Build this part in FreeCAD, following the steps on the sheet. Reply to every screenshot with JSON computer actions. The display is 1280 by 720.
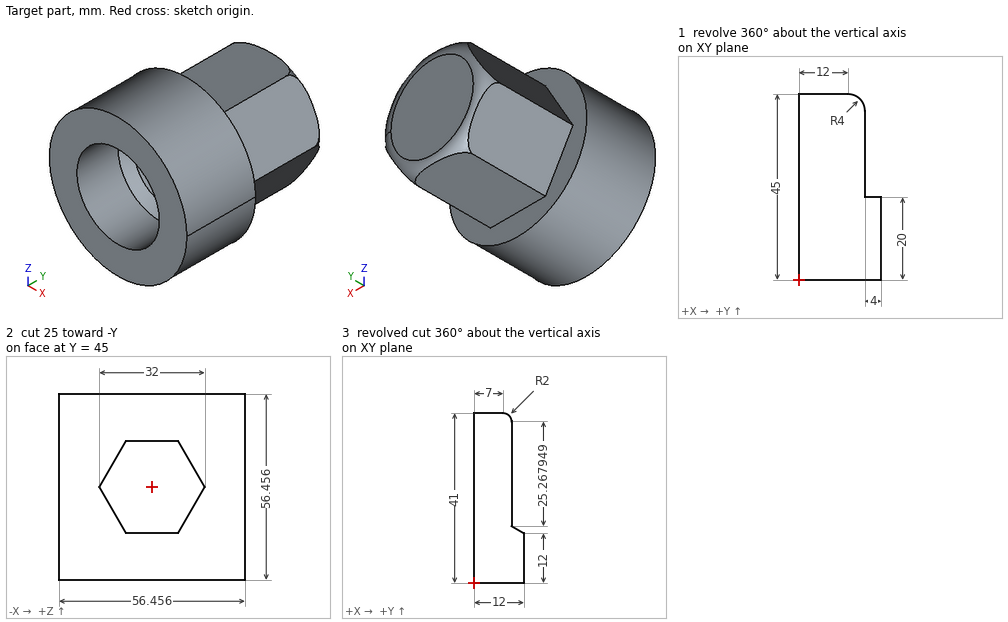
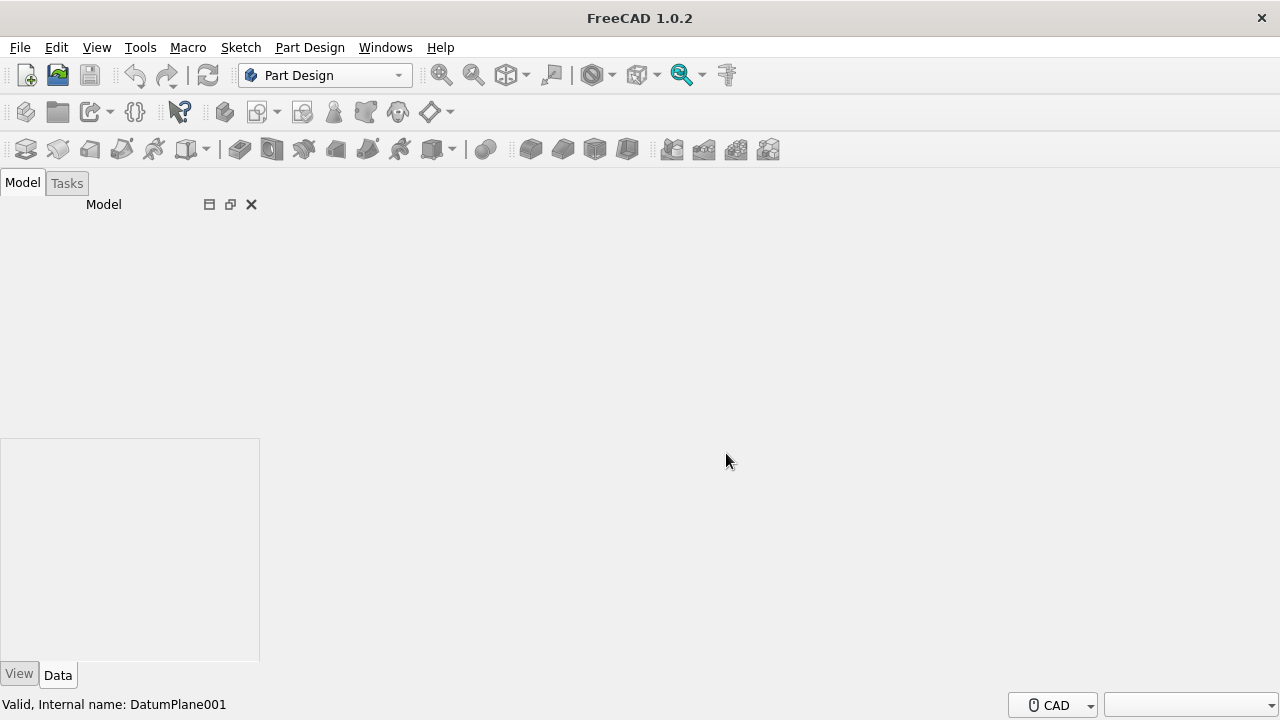
{"action": "key", "text": "ctrl+n"}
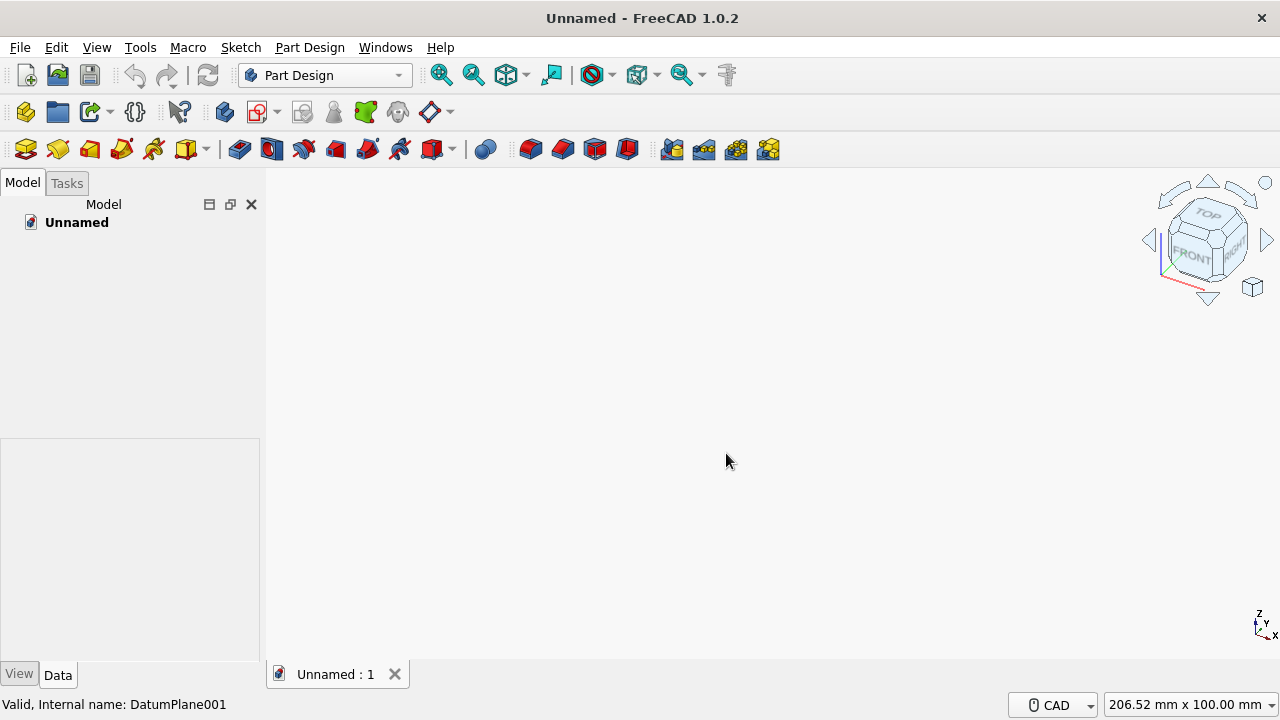
{"action": "left_click", "coordinate": [258, 112]}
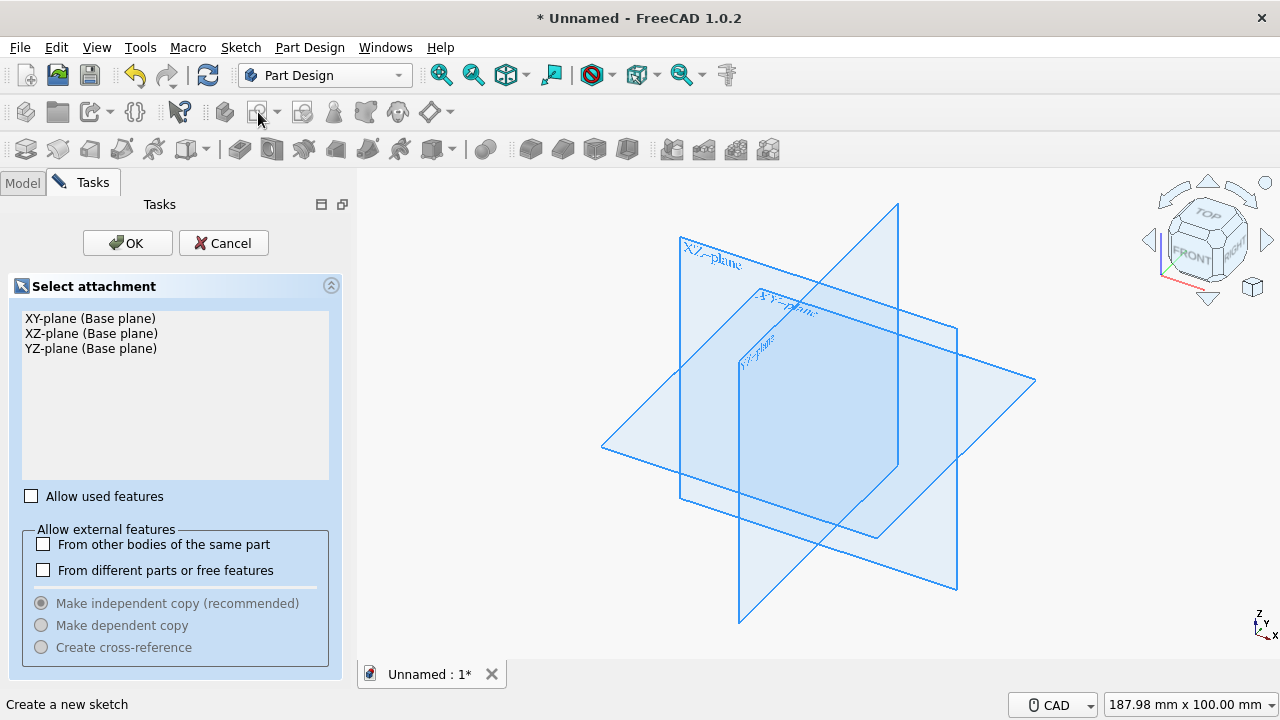
{"action": "left_click", "coordinate": [82, 318]}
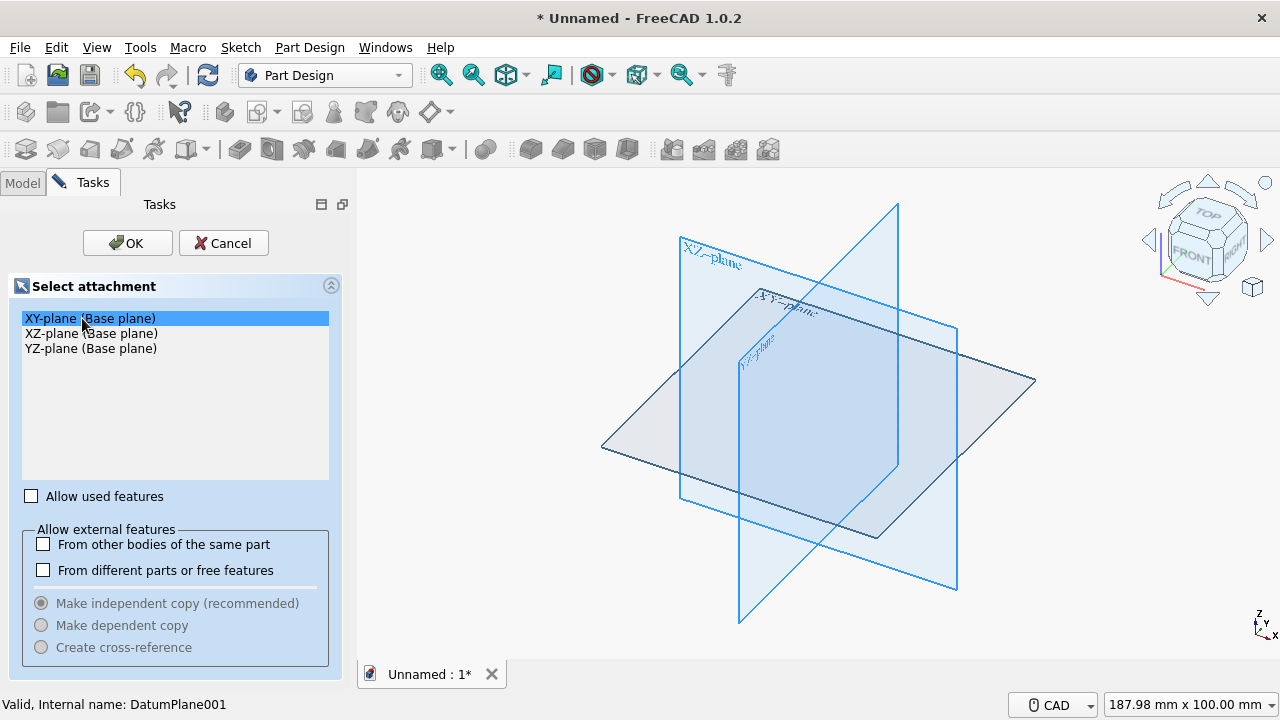
{"action": "left_click", "coordinate": [128, 243]}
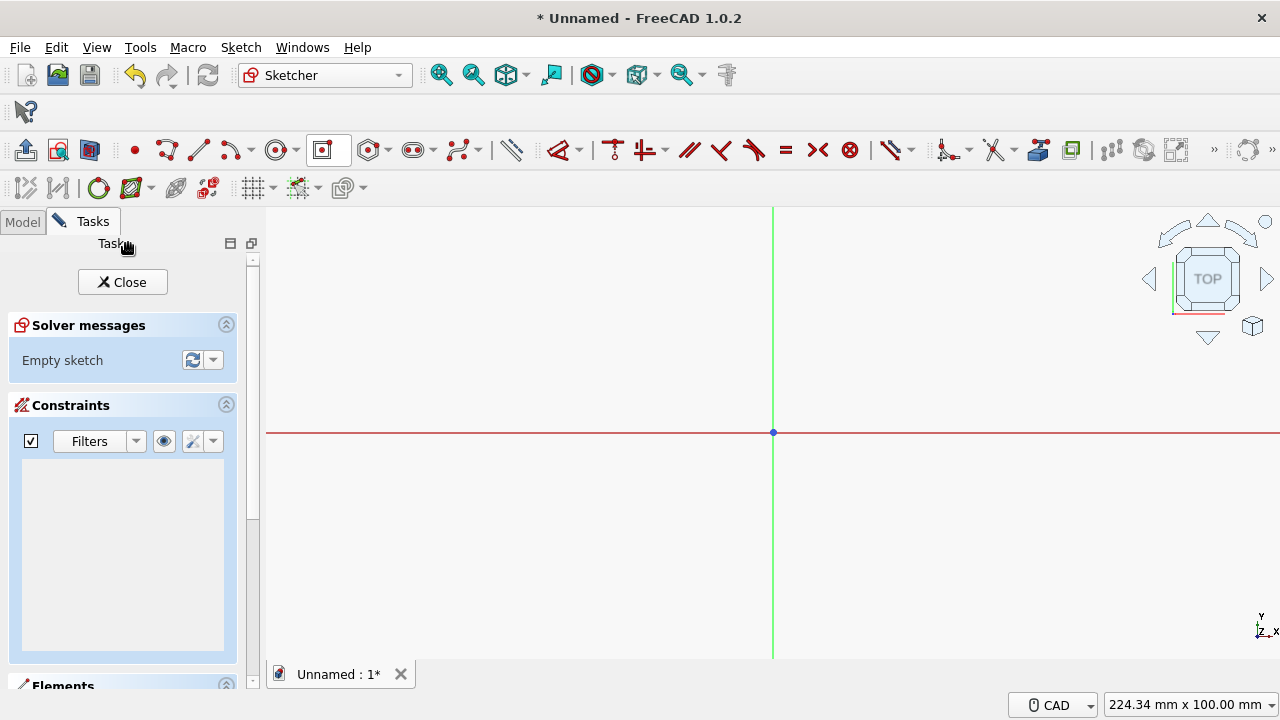
{"action": "scroll", "coordinate": [294, 631], "scroll_direction": "down", "scroll_amount": 1}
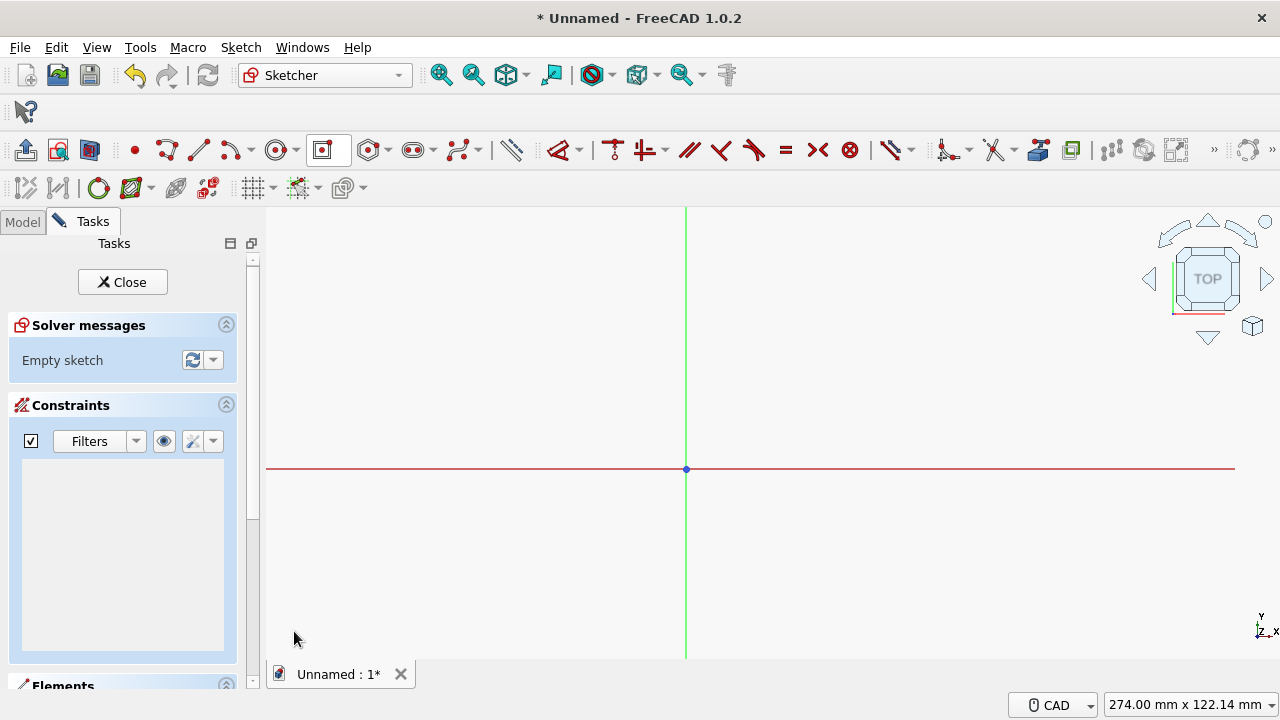
{"action": "scroll", "coordinate": [746, 328], "scroll_direction": "up", "scroll_amount": 3}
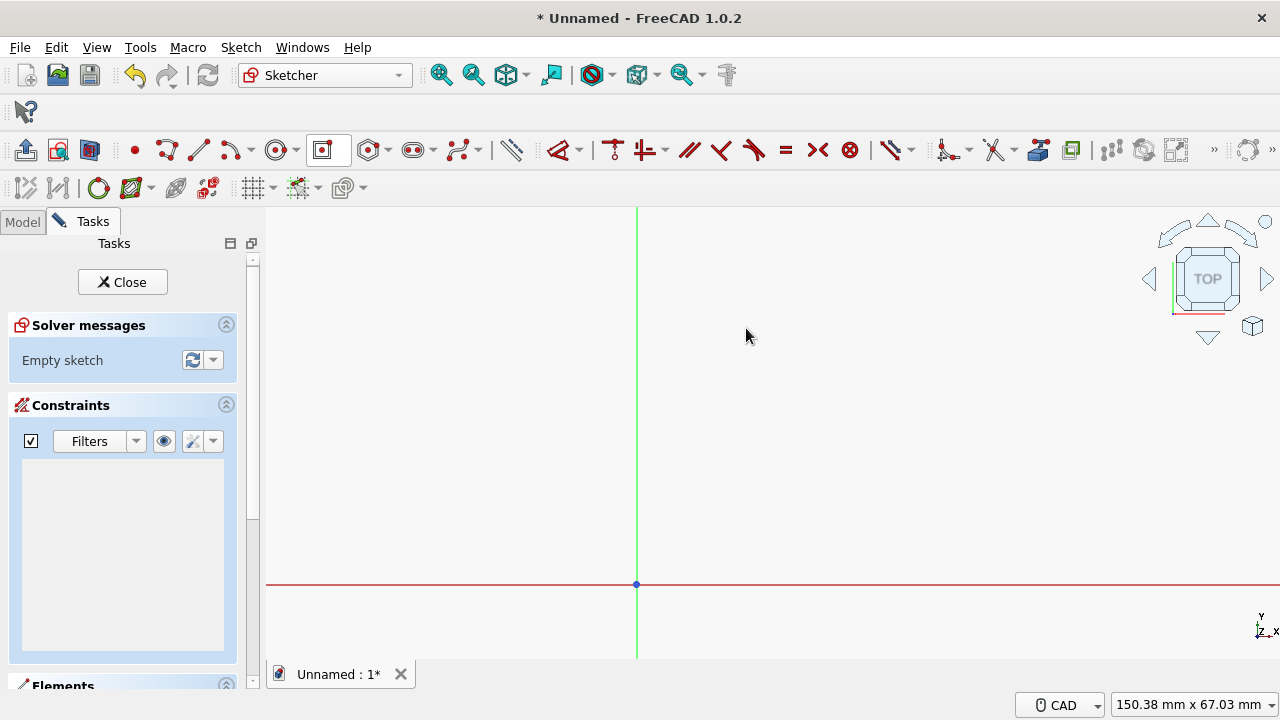
{"action": "key", "text": "g m"}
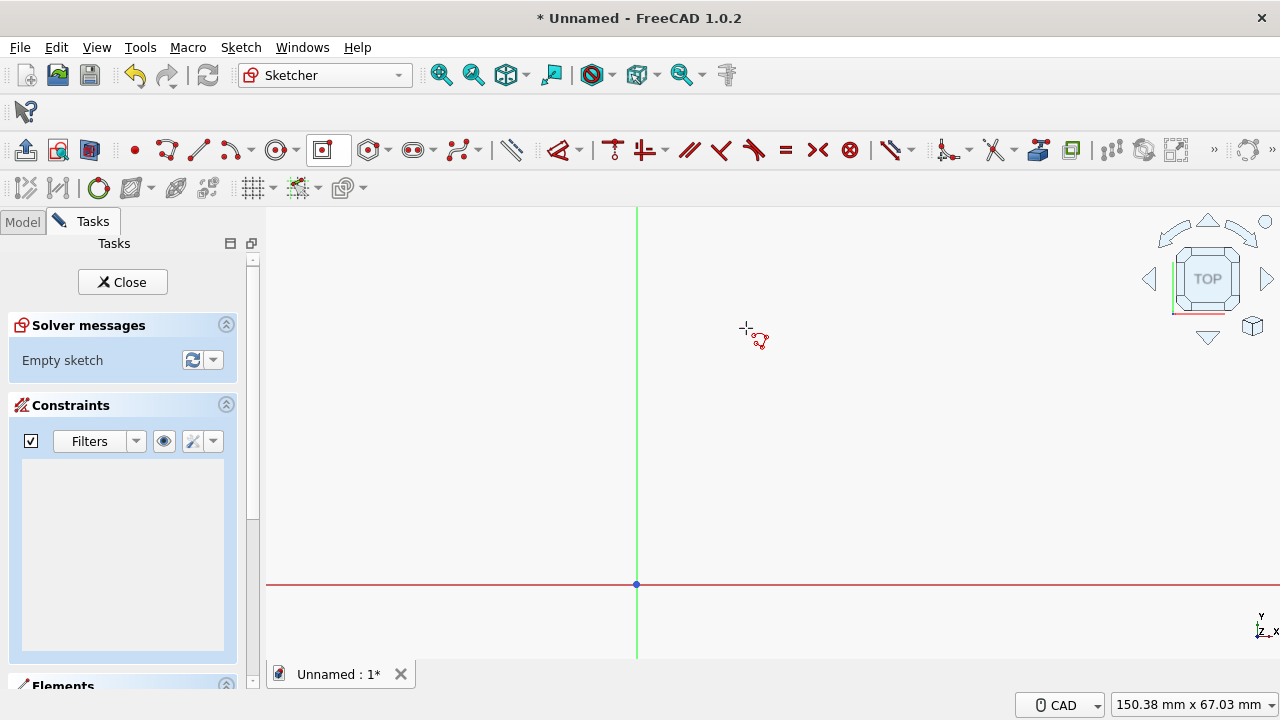
{"action": "left_click", "coordinate": [718, 281]}
{"action": "left_click", "coordinate": [637, 281]}
{"action": "left_click", "coordinate": [637, 585]}
{"action": "left_click", "coordinate": [771, 576]}
{"action": "left_click", "coordinate": [771, 450]}
{"action": "left_click", "coordinate": [744, 450]}
{"action": "left_click", "coordinate": [744, 308]}
{"action": "right_click", "coordinate": [744, 308]}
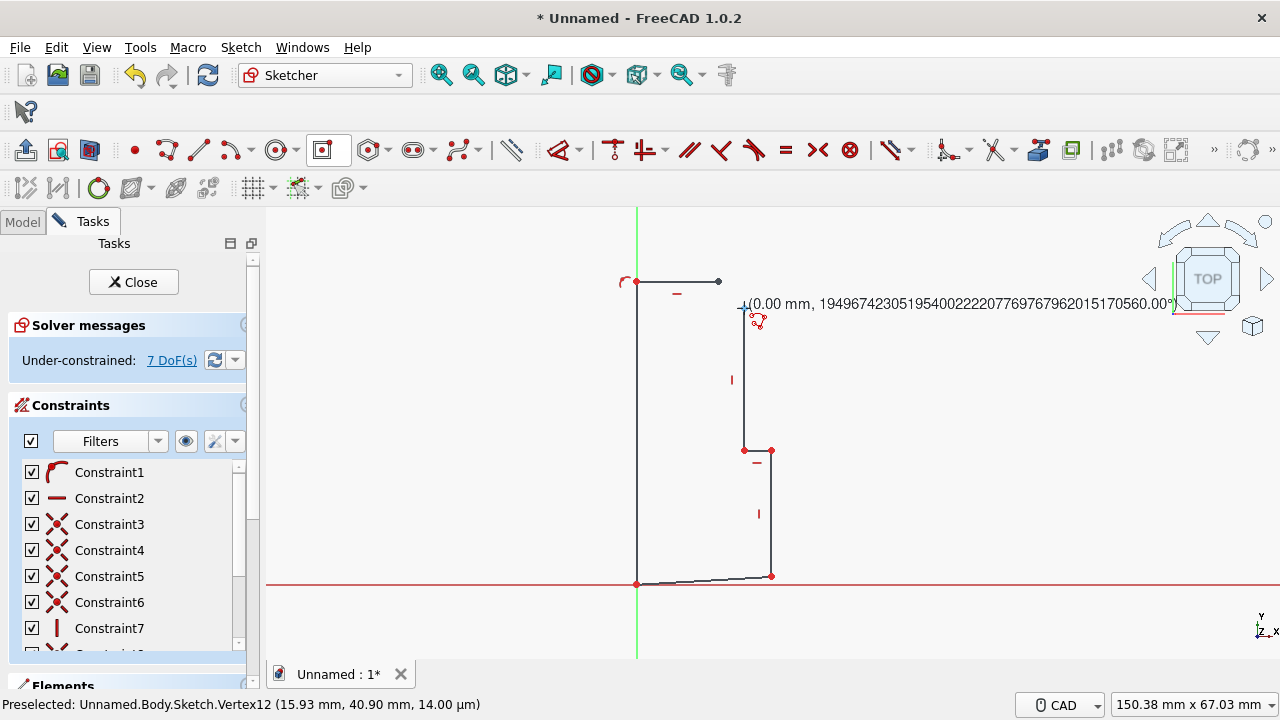
{"action": "key", "text": "g 3 a"}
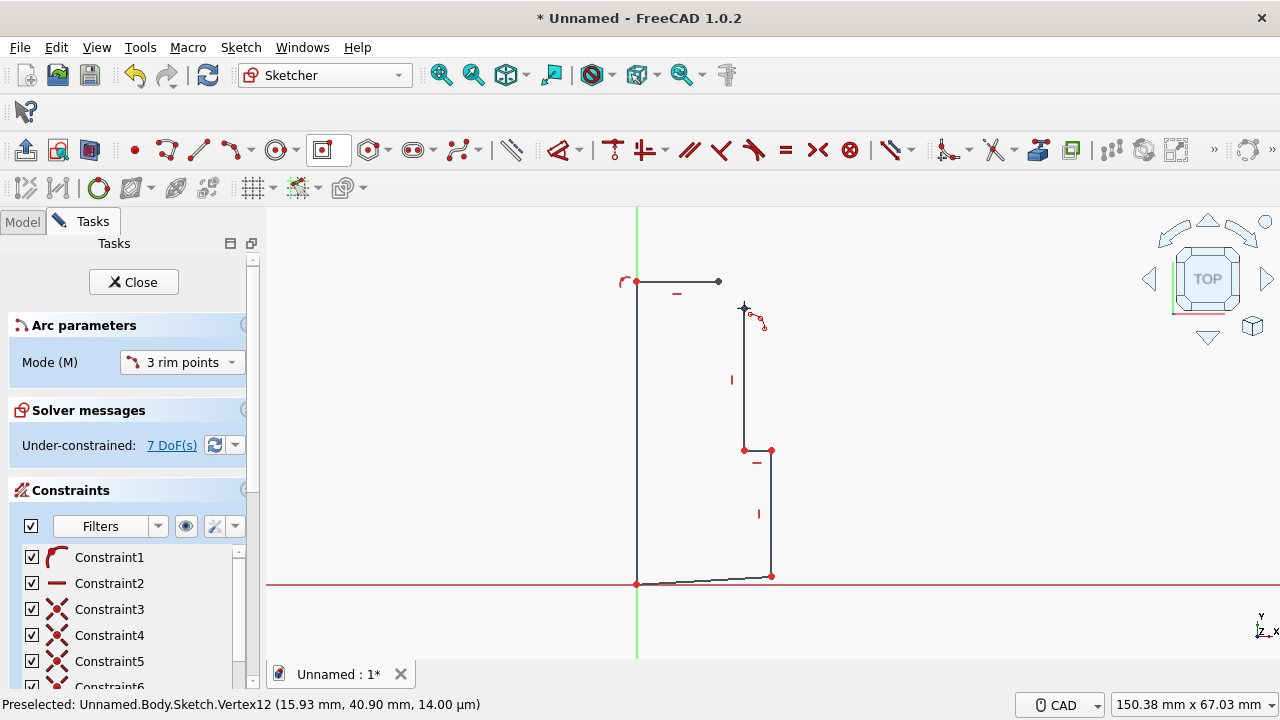
{"action": "left_click", "coordinate": [744, 309]}
{"action": "left_click", "coordinate": [718, 282]}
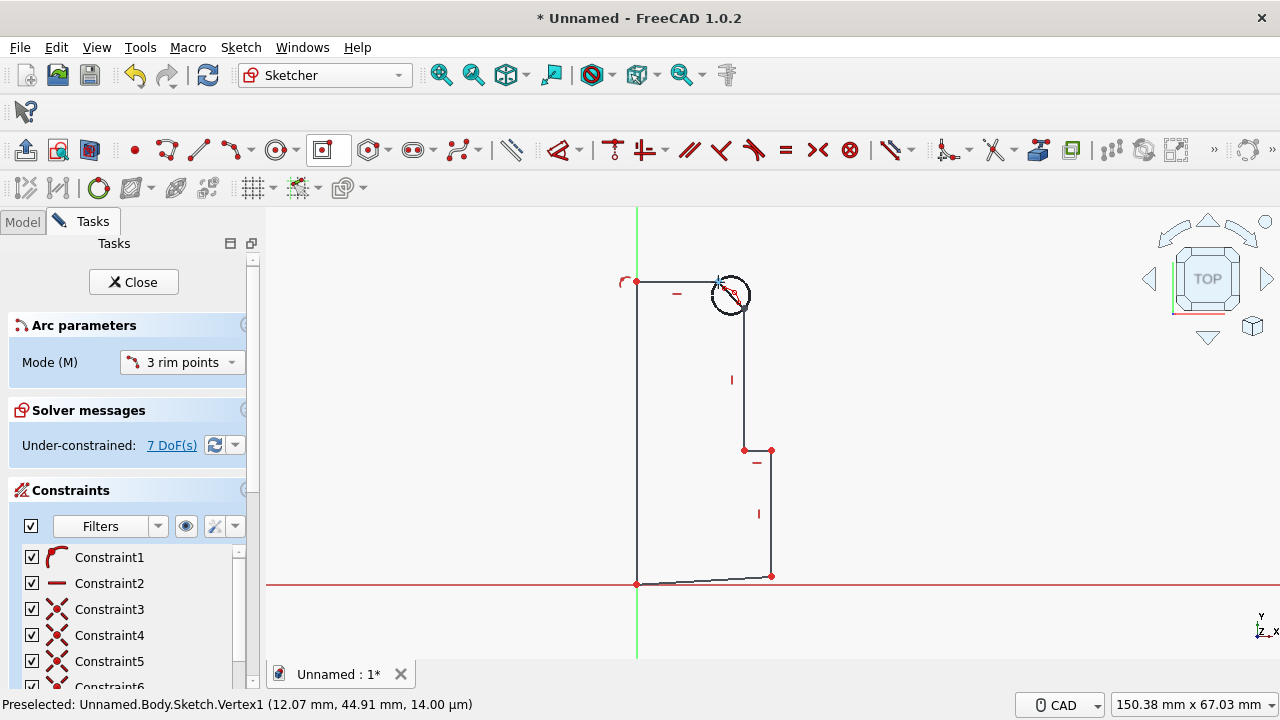
{"action": "scroll", "coordinate": [737, 289], "scroll_direction": "up", "scroll_amount": 4}